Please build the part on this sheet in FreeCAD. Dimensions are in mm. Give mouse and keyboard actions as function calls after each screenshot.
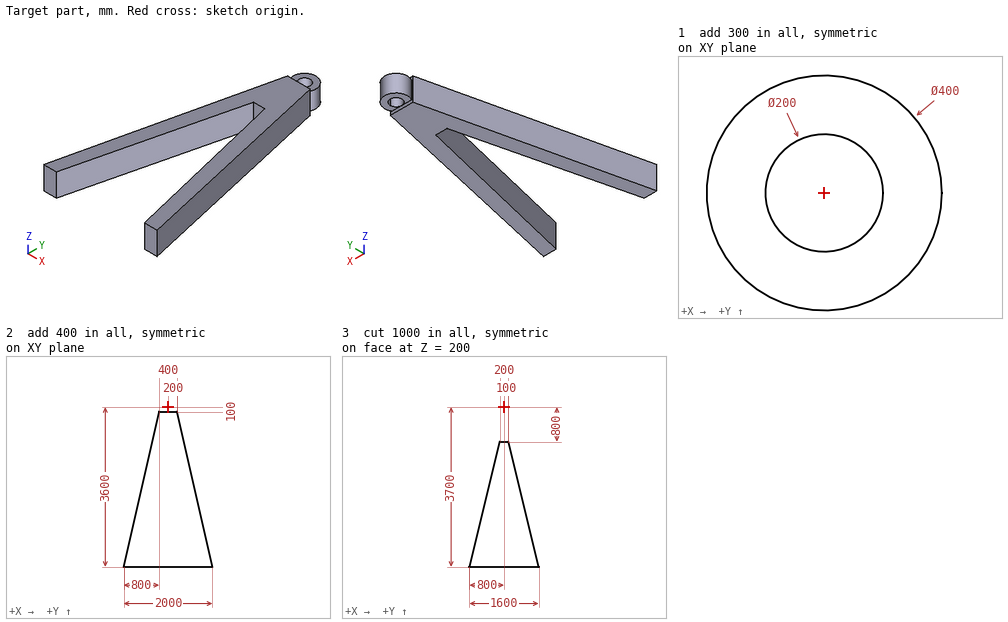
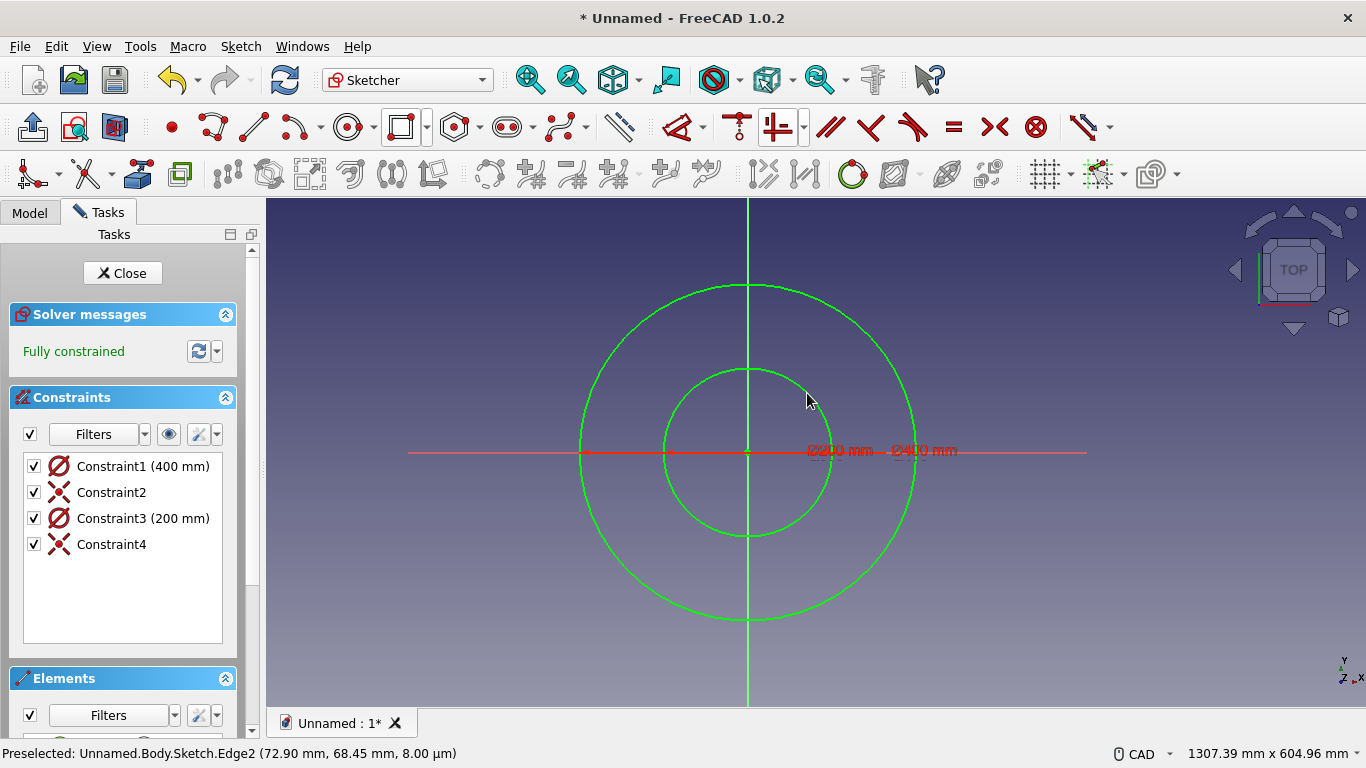
click(123, 273)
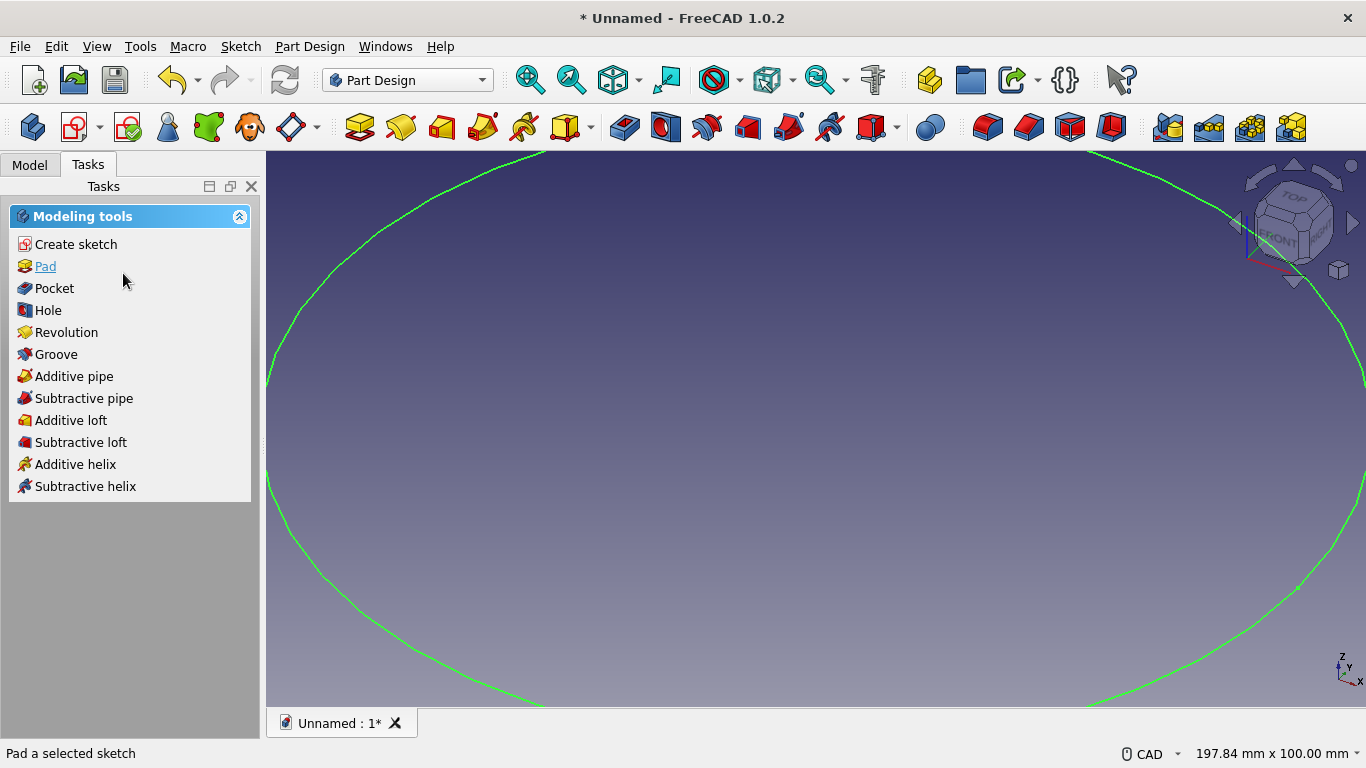
click(360, 128)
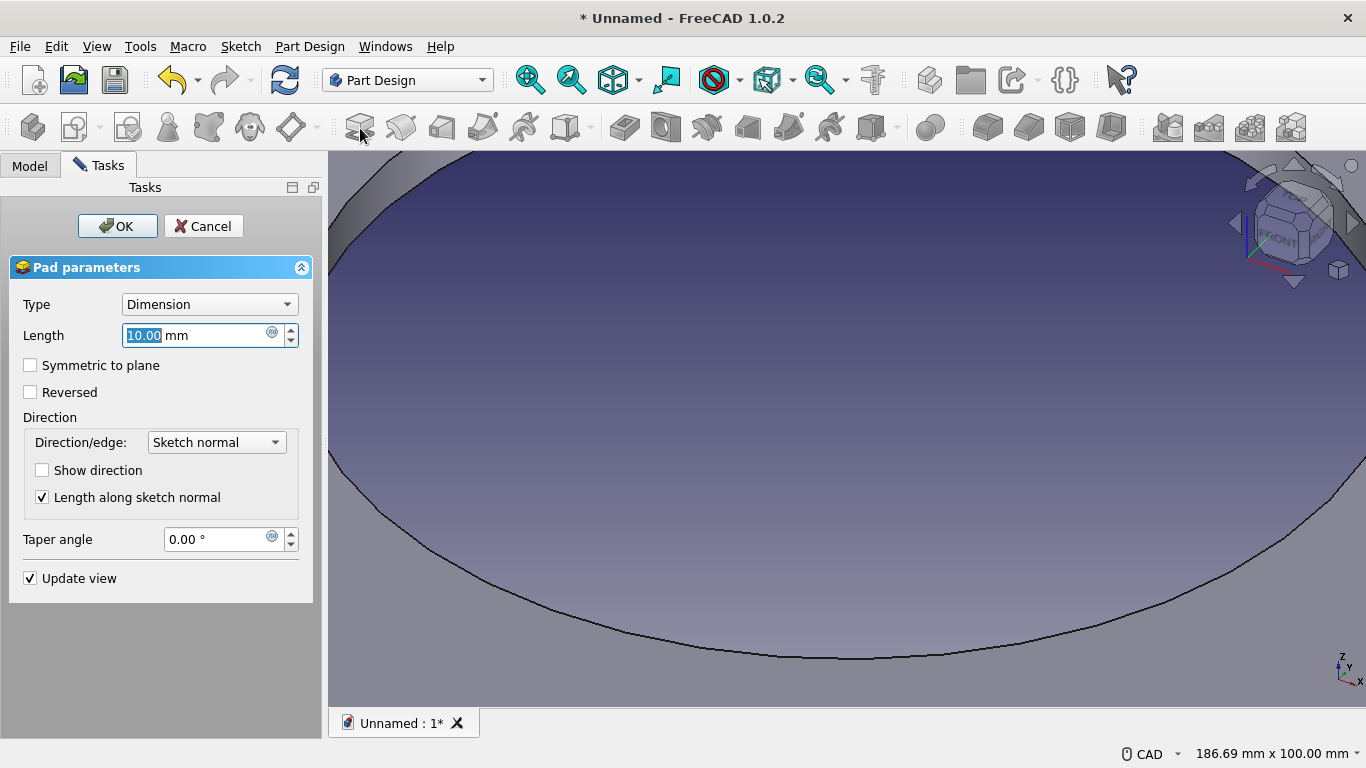
text(300)
key(Tab)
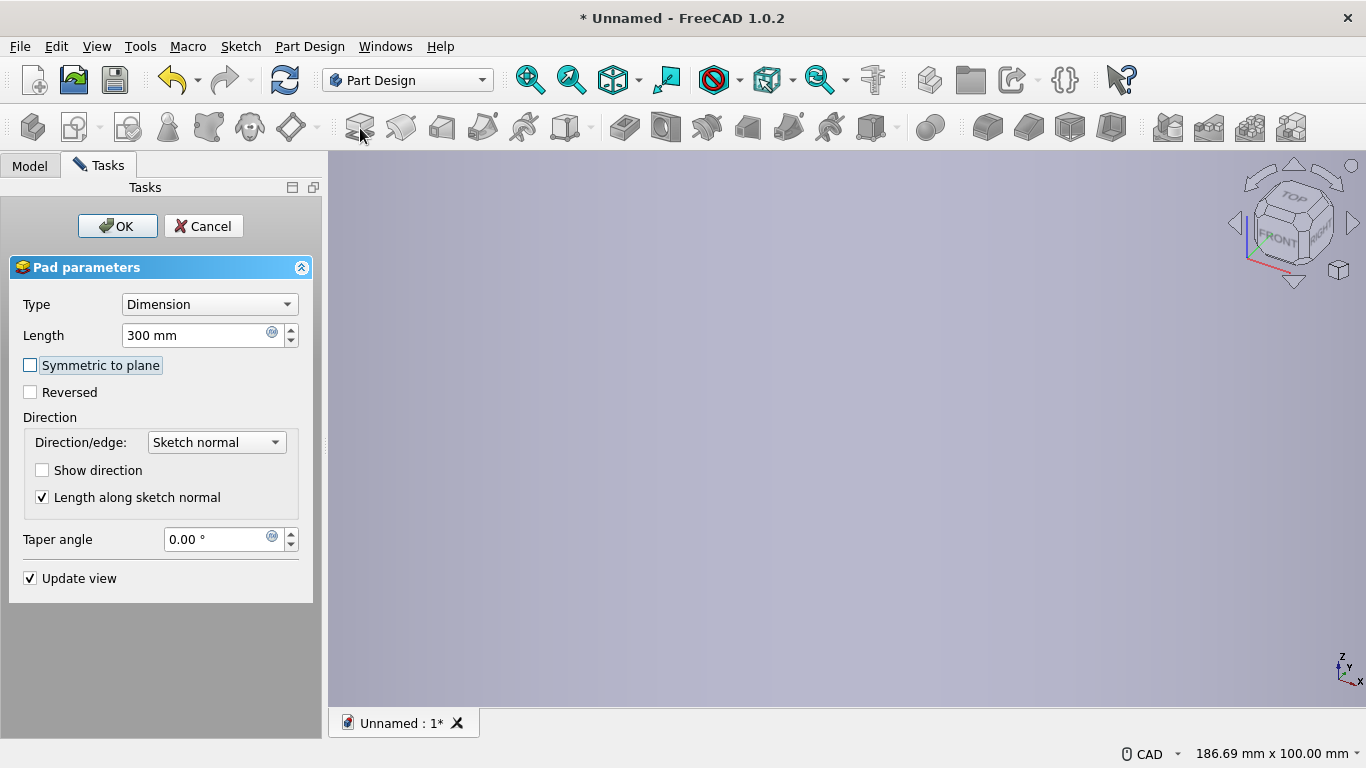
click(31, 365)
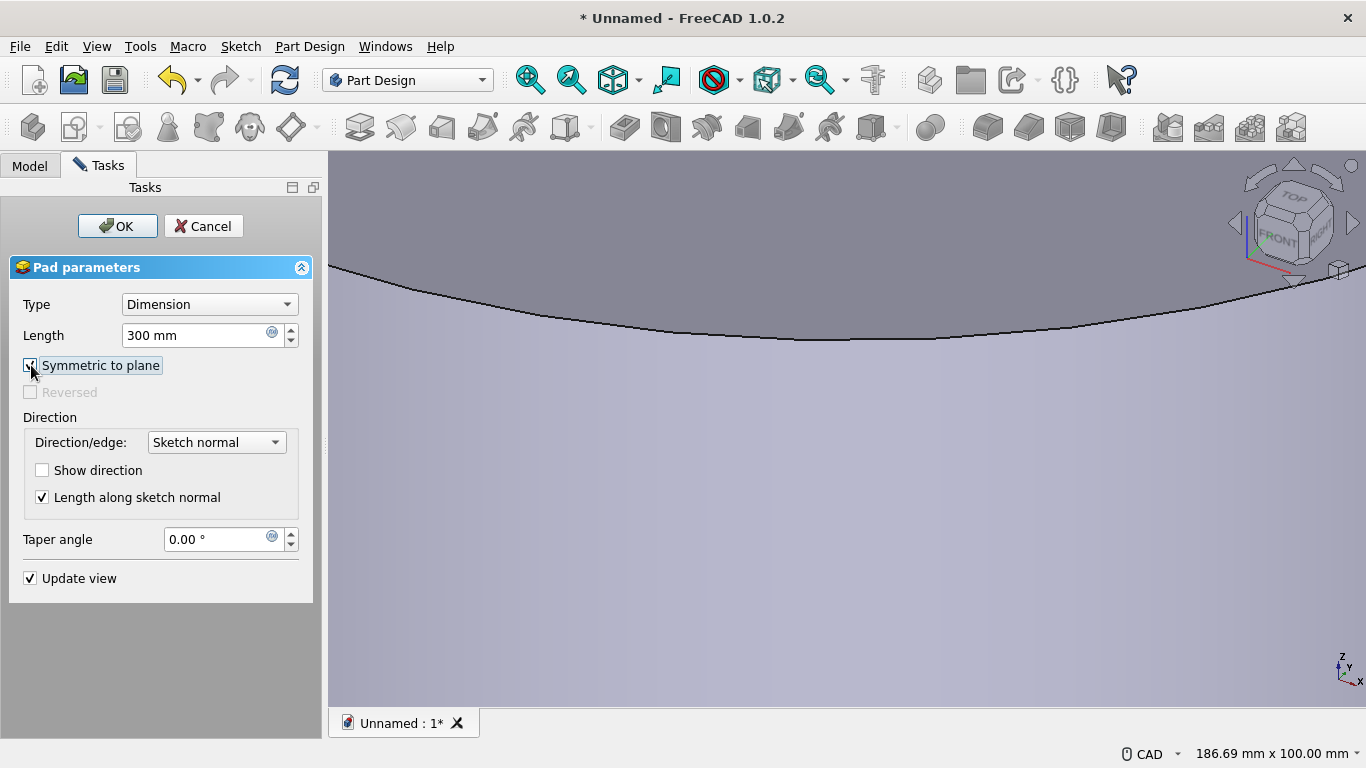
click(118, 226)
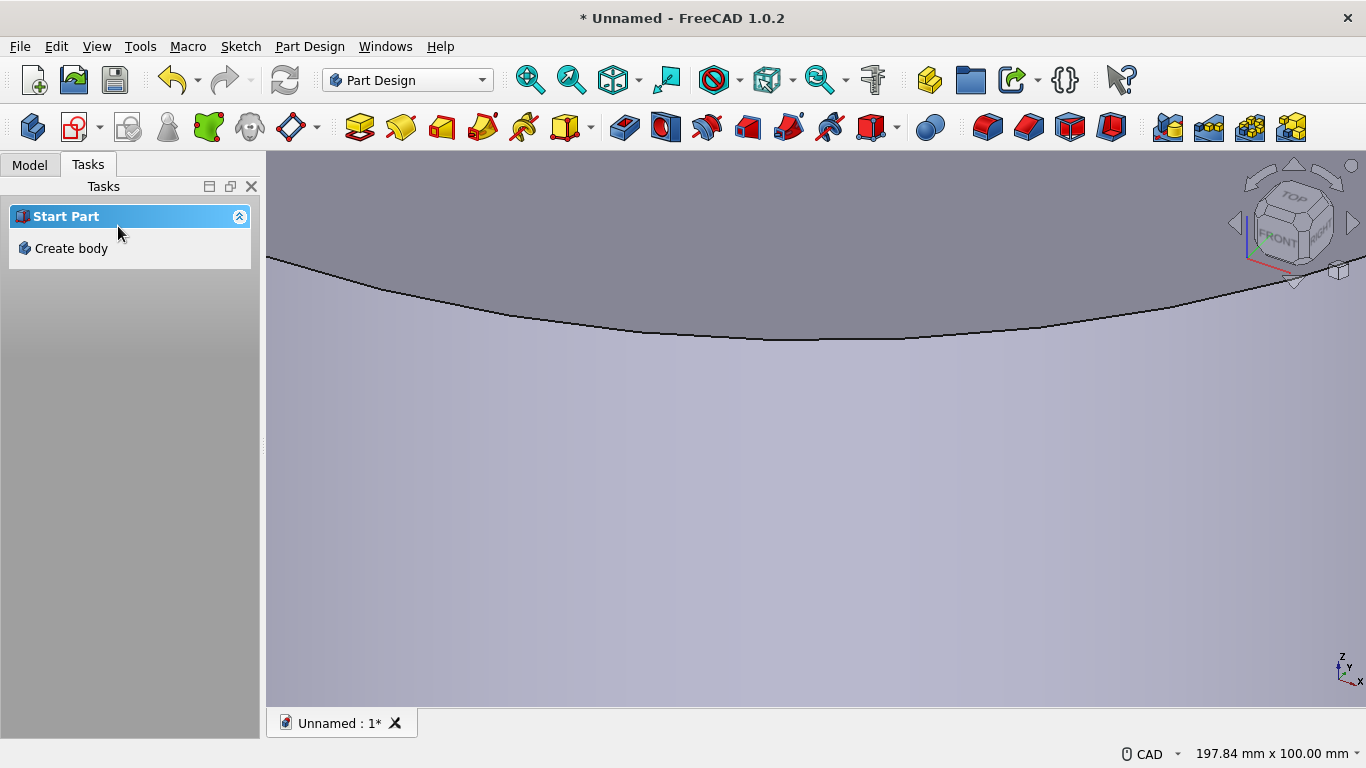
click(531, 80)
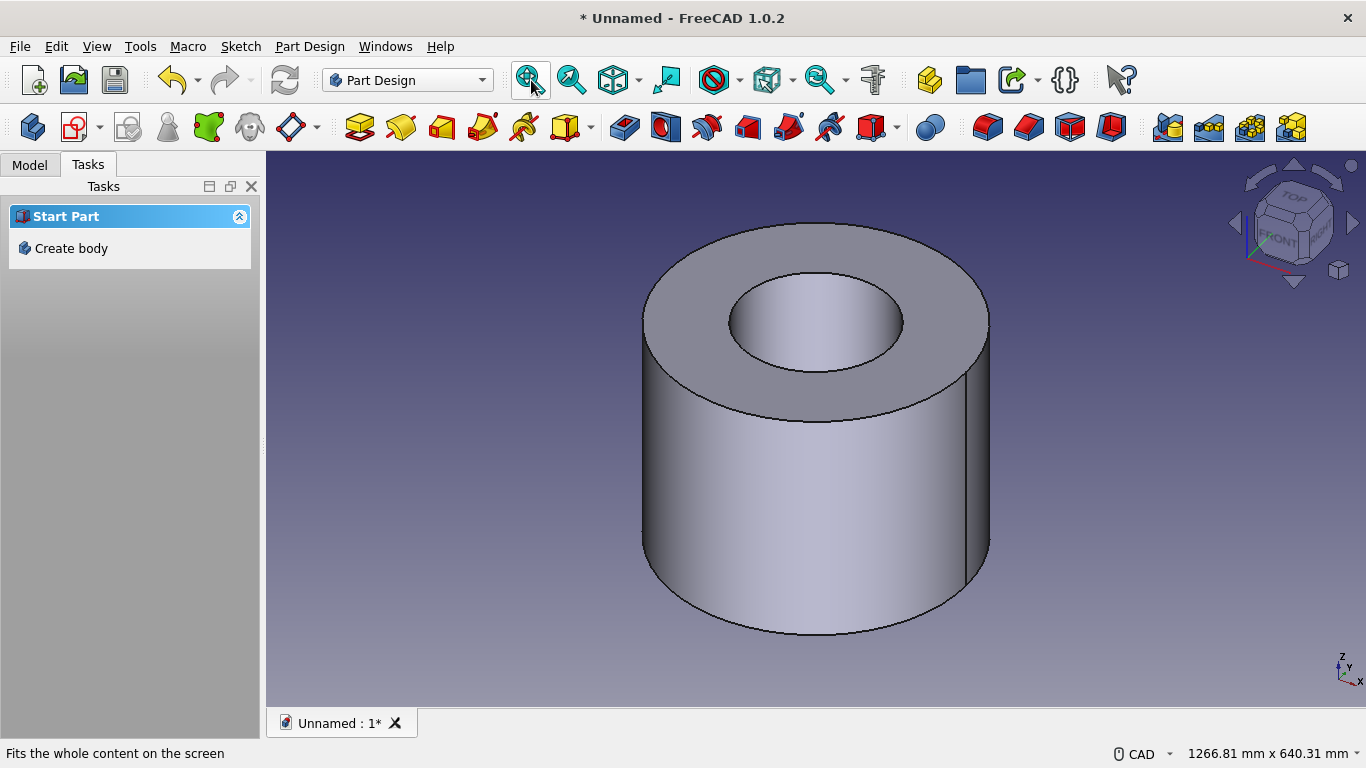
click(74, 128)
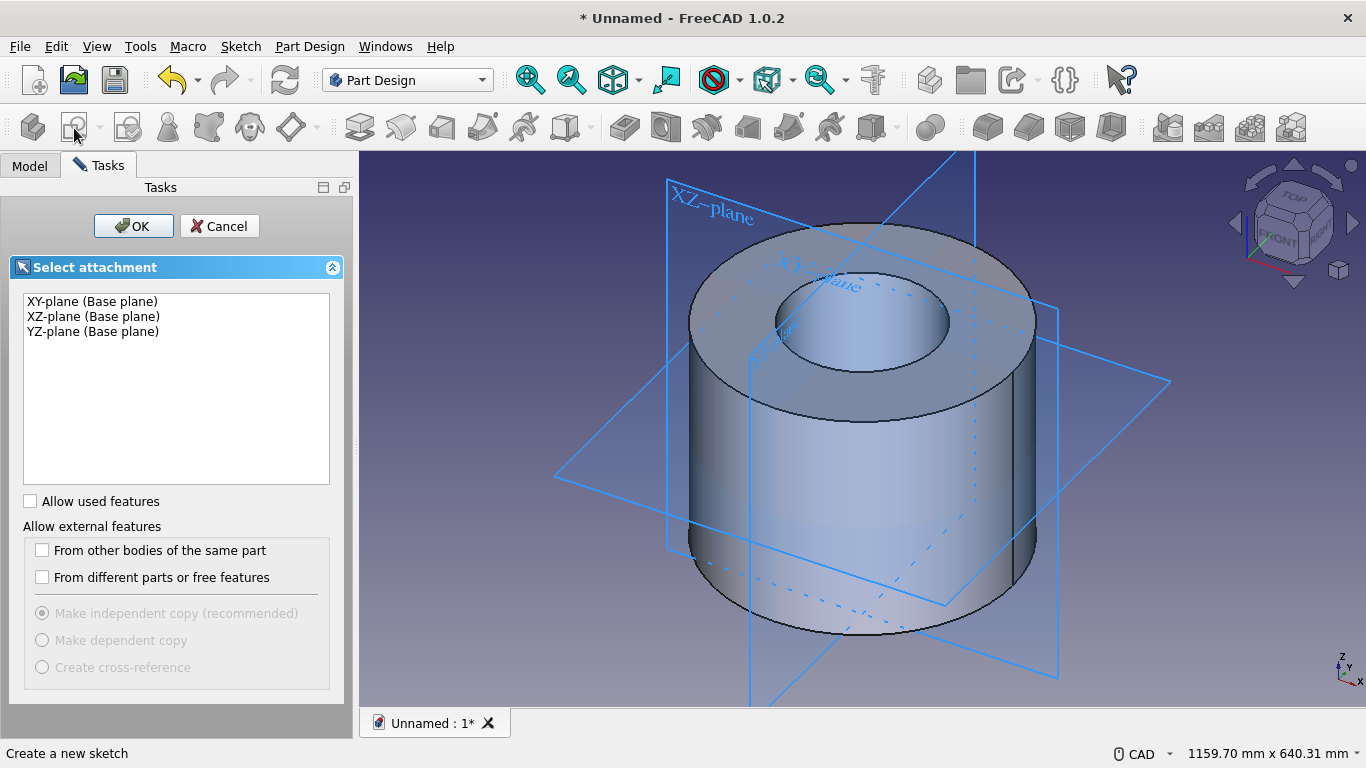
click(84, 302)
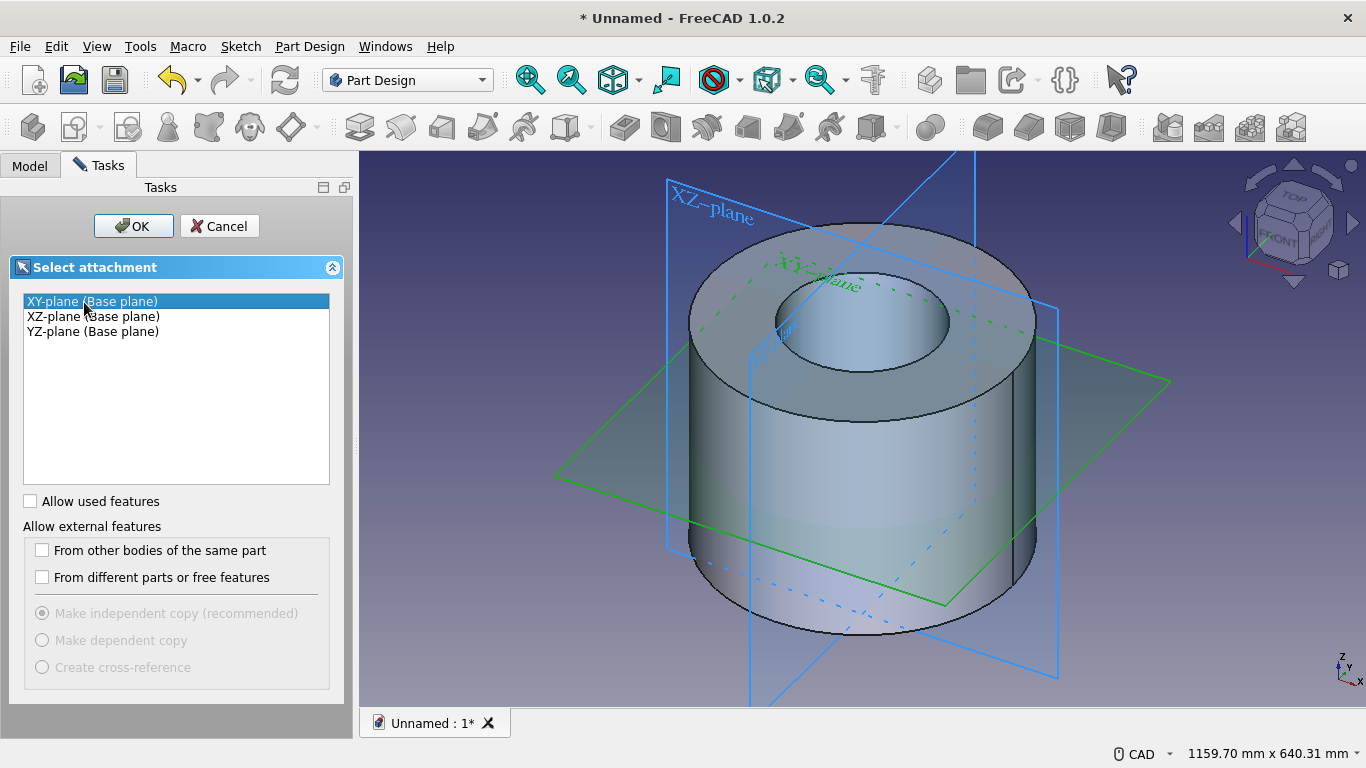
click(134, 226)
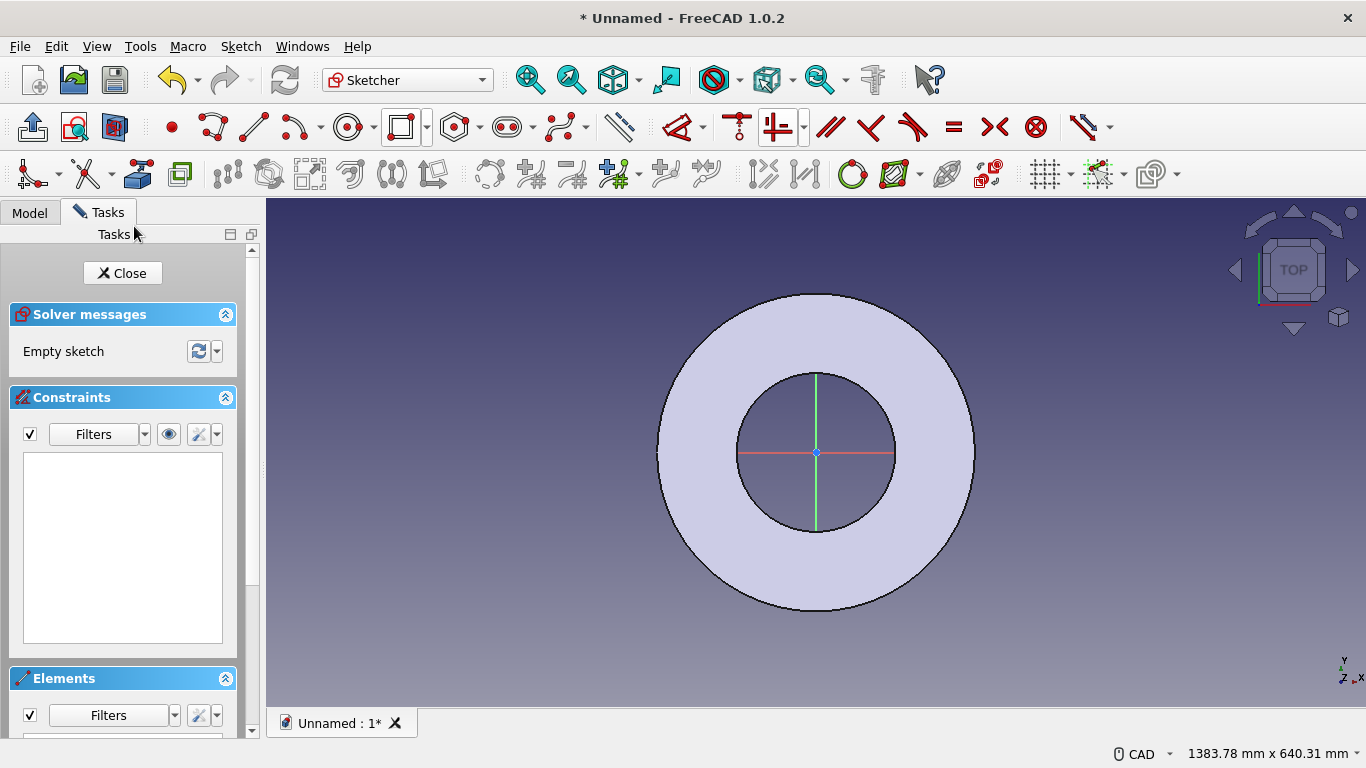
click(115, 128)